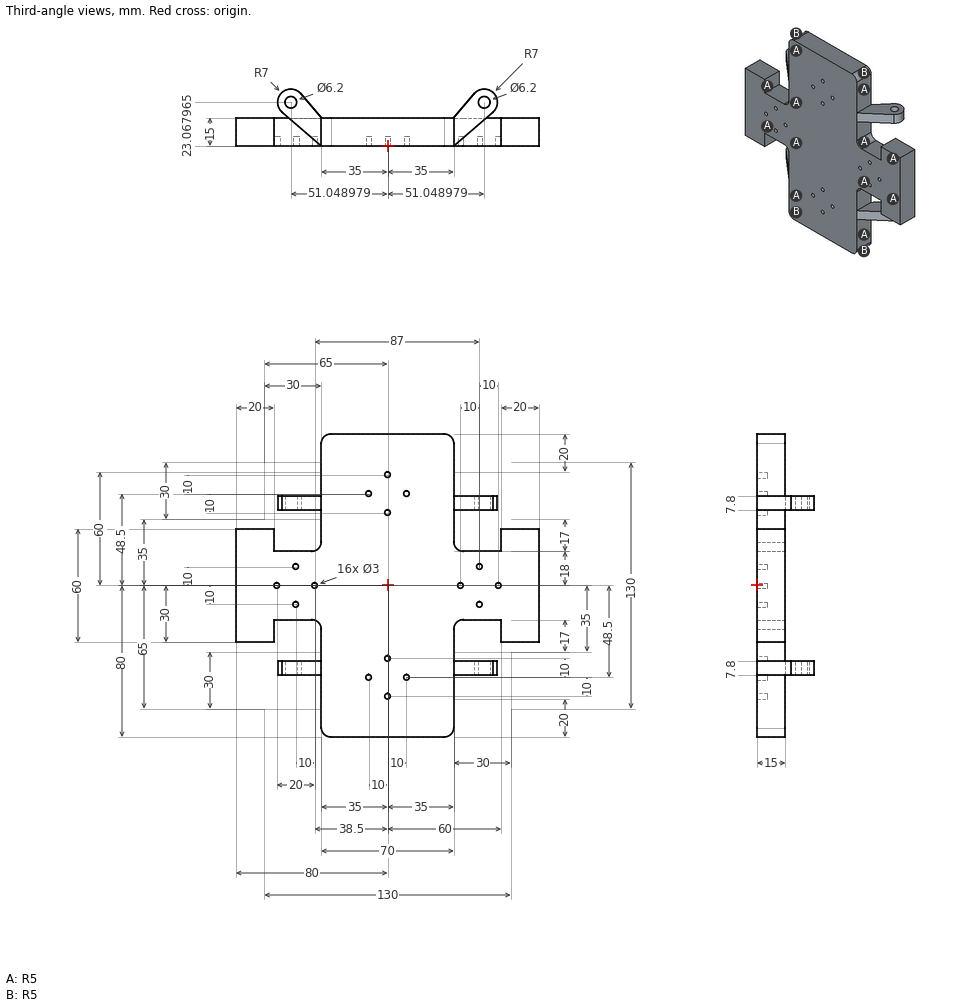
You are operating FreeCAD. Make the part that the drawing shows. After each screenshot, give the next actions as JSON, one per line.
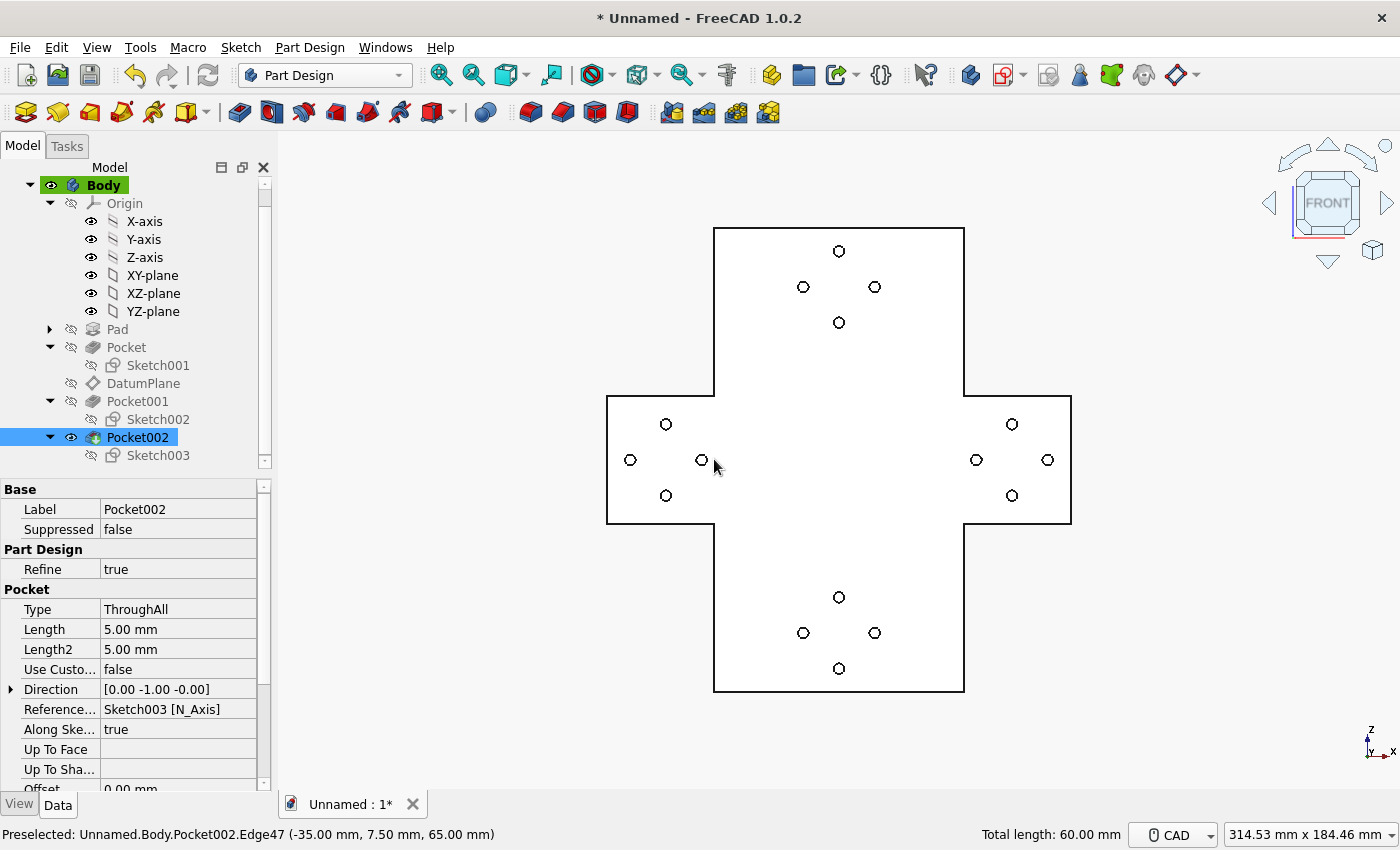
{"action": "key", "text": "3"}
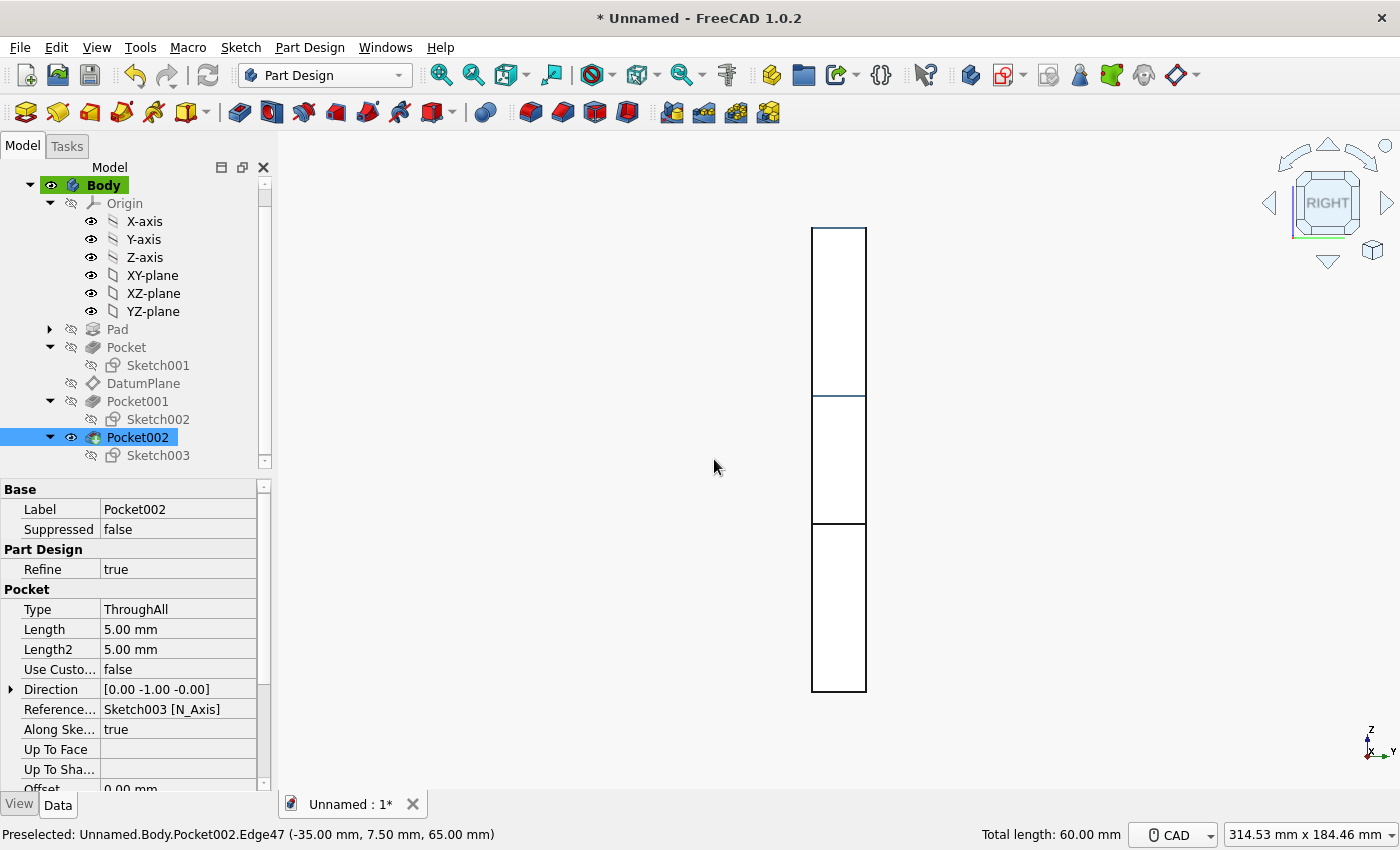
{"action": "left_click", "coordinate": [839, 523], "text": "ctrl"}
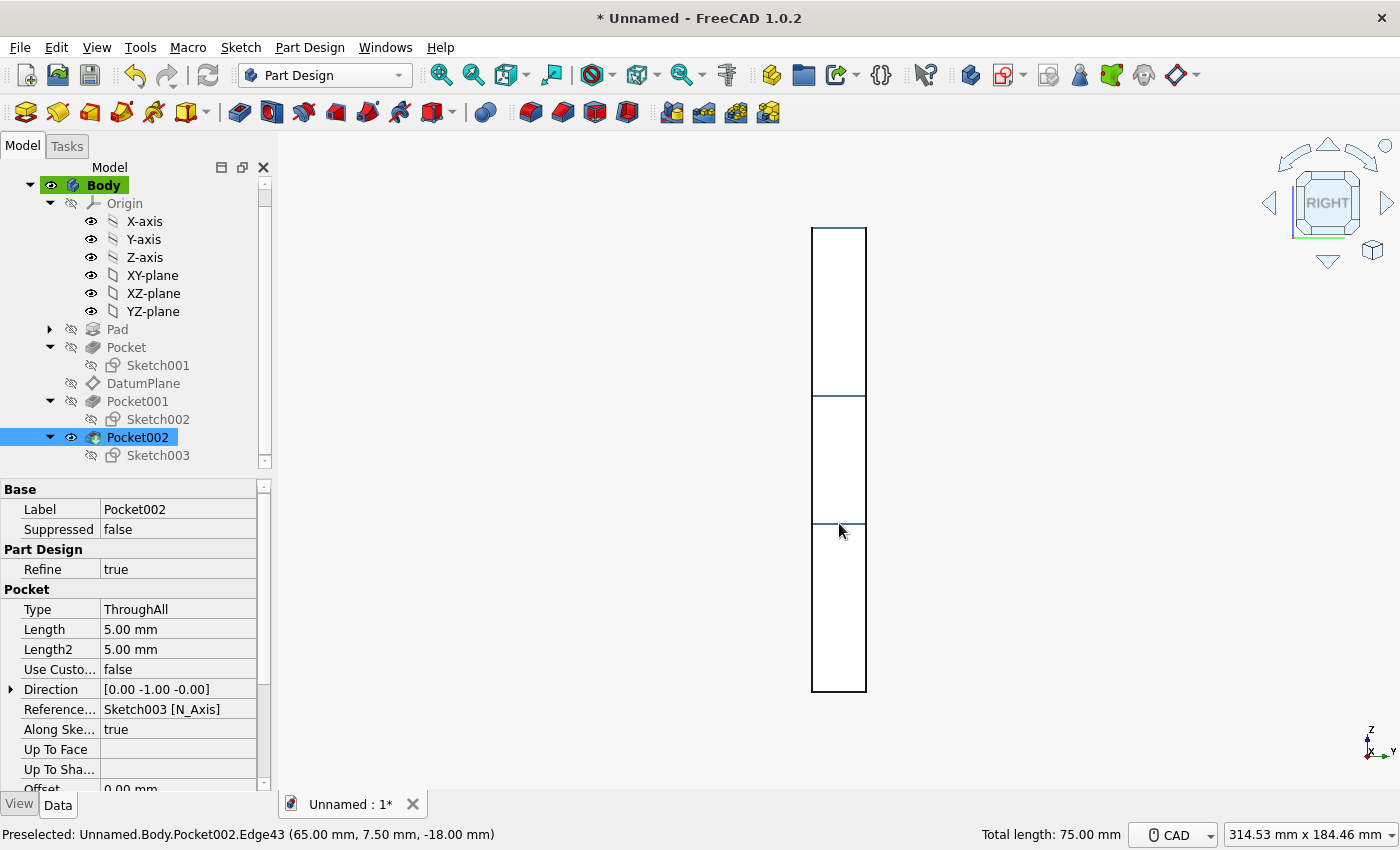
{"action": "left_click", "coordinate": [839, 691], "text": "ctrl"}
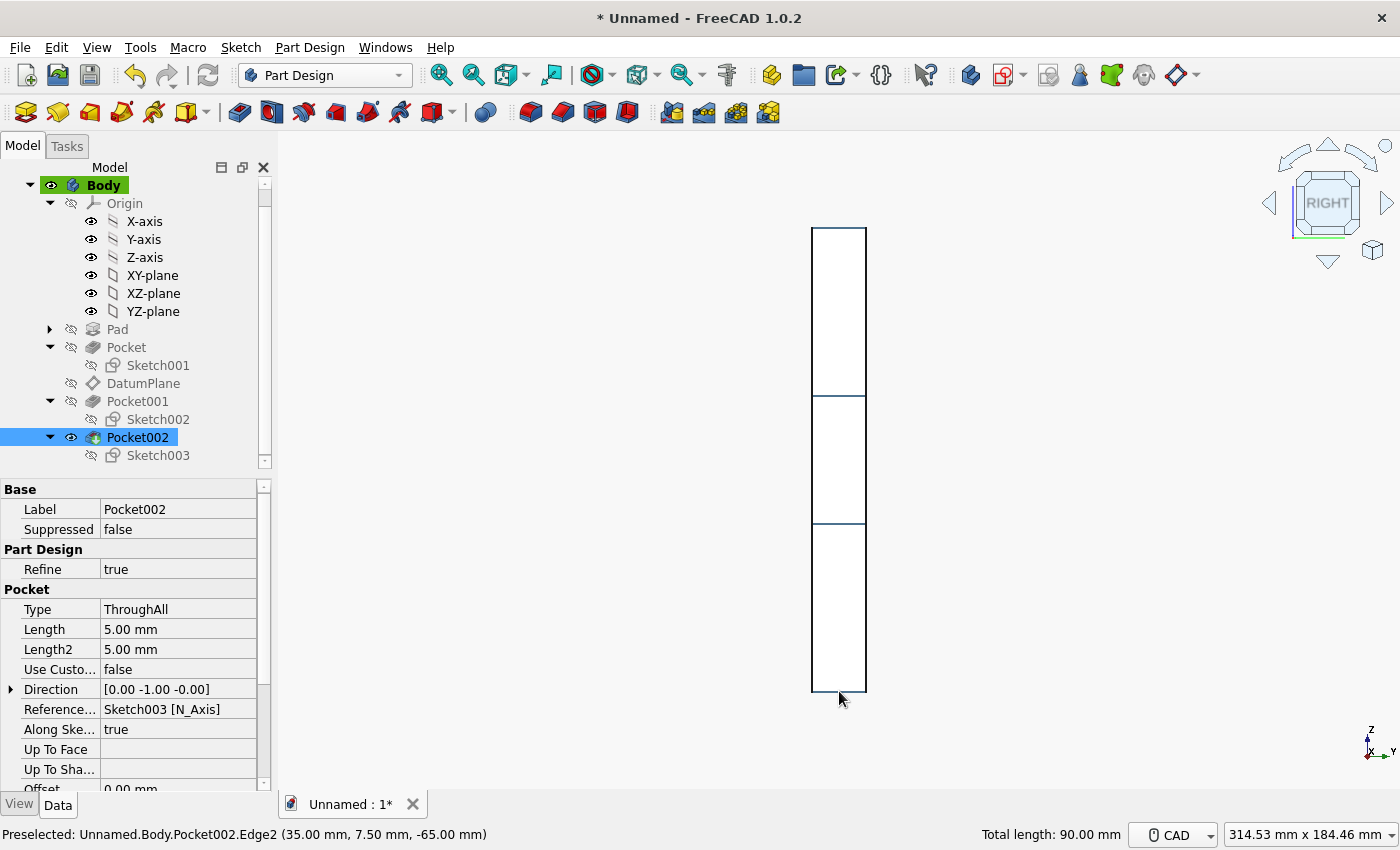
{"action": "key", "text": "5"}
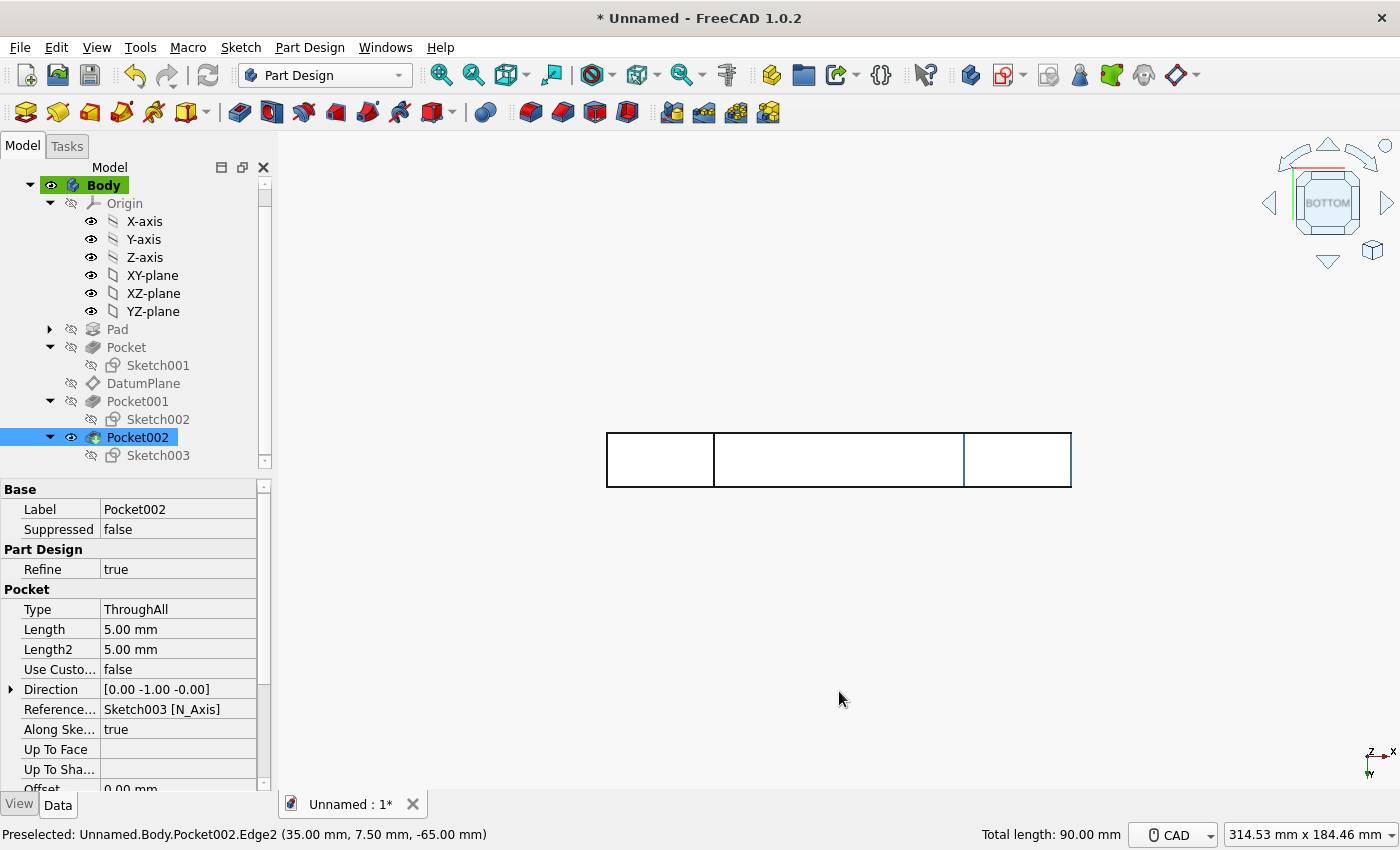
{"action": "left_click", "coordinate": [442, 76]}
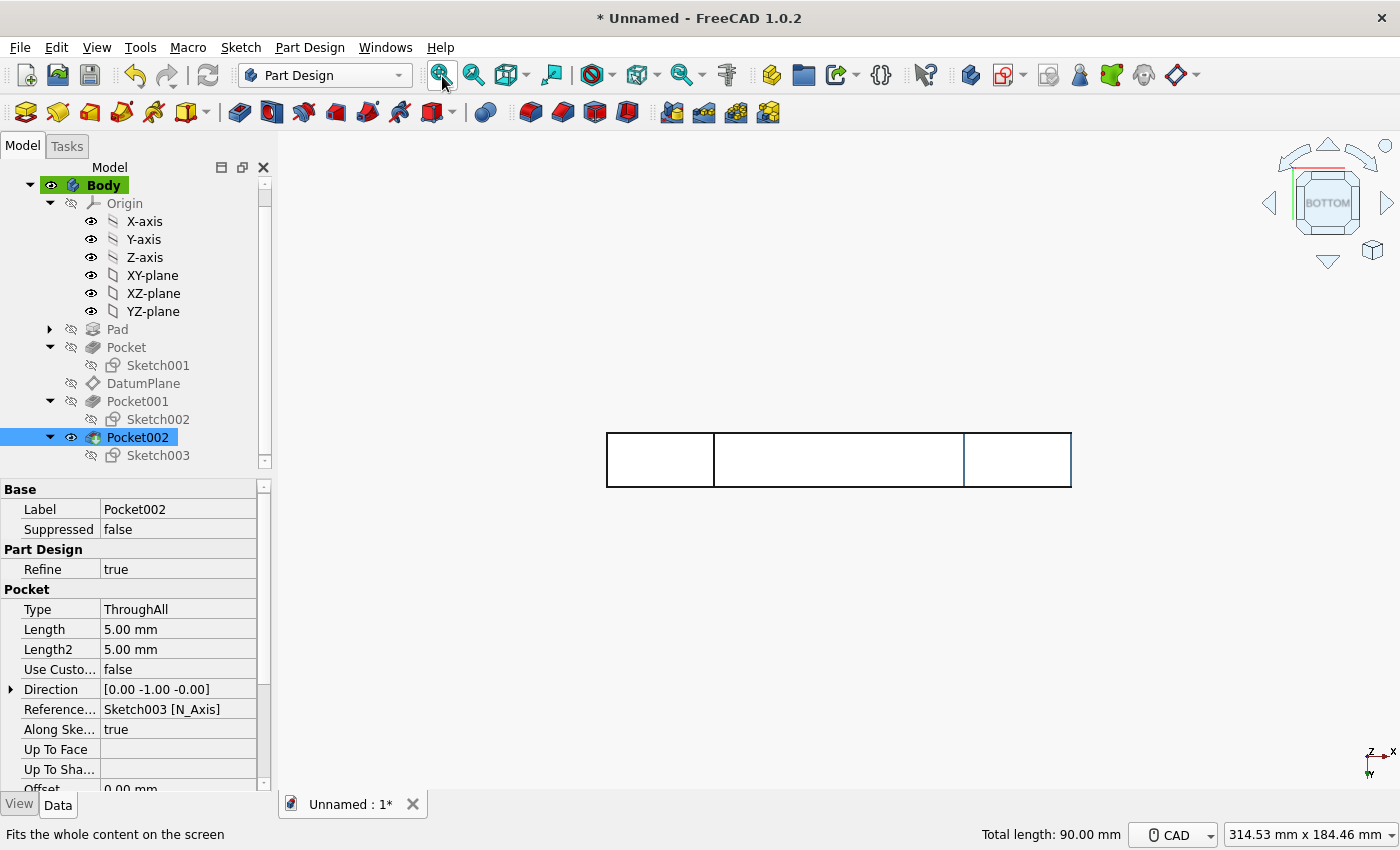
{"action": "left_click", "coordinate": [607, 459], "text": "ctrl"}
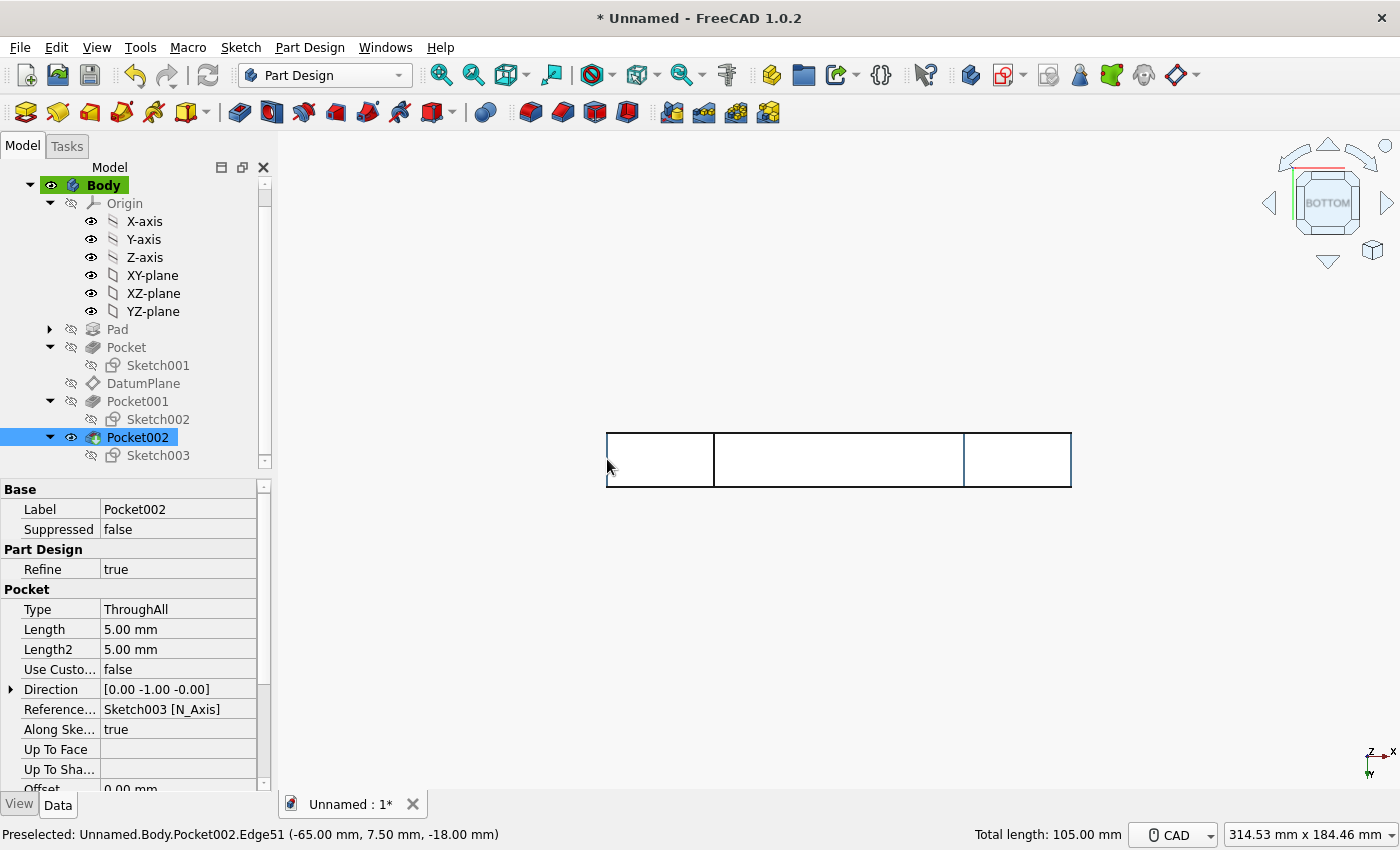
{"action": "left_click", "coordinate": [714, 459], "text": "ctrl"}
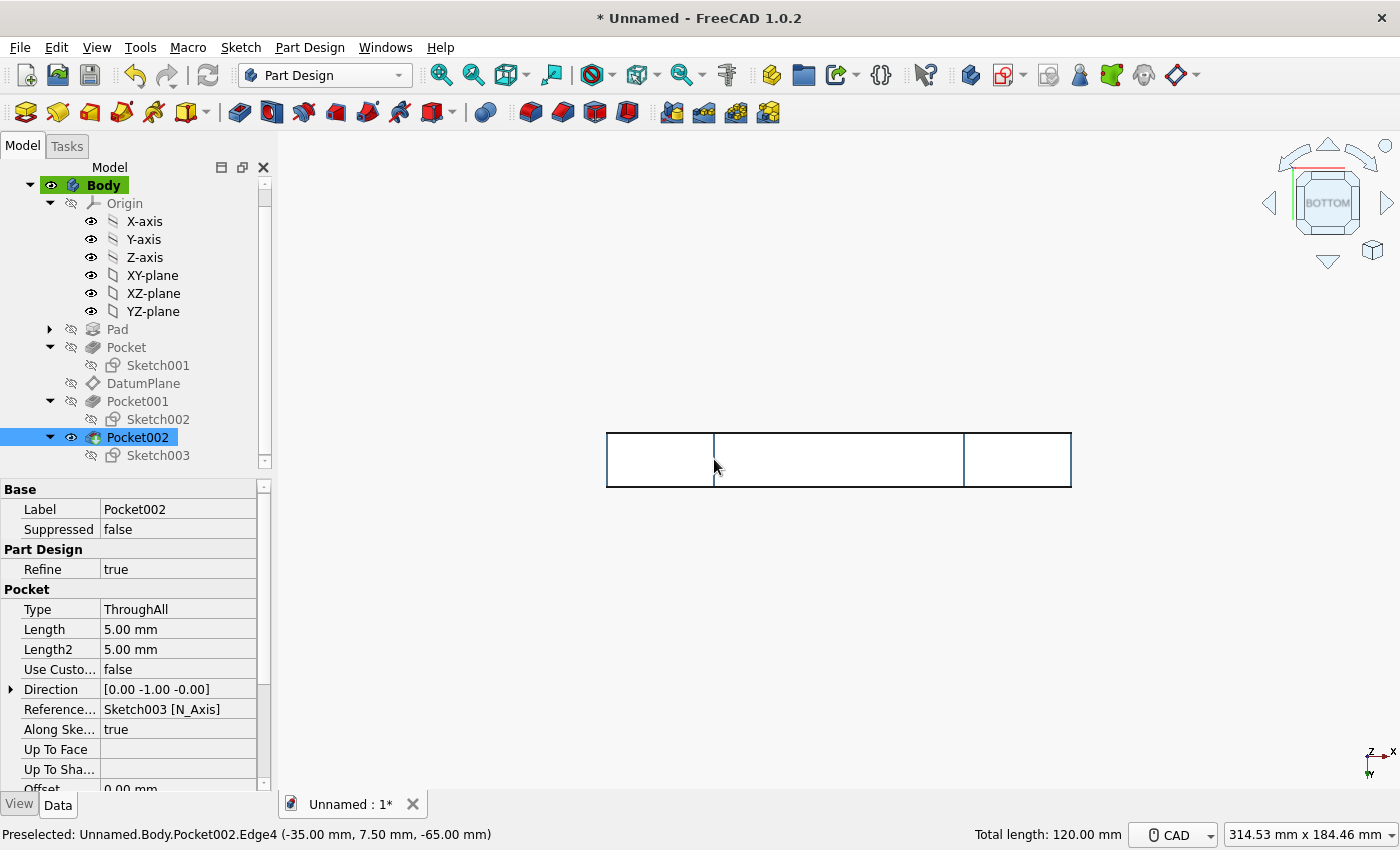
{"action": "key", "text": "4"}